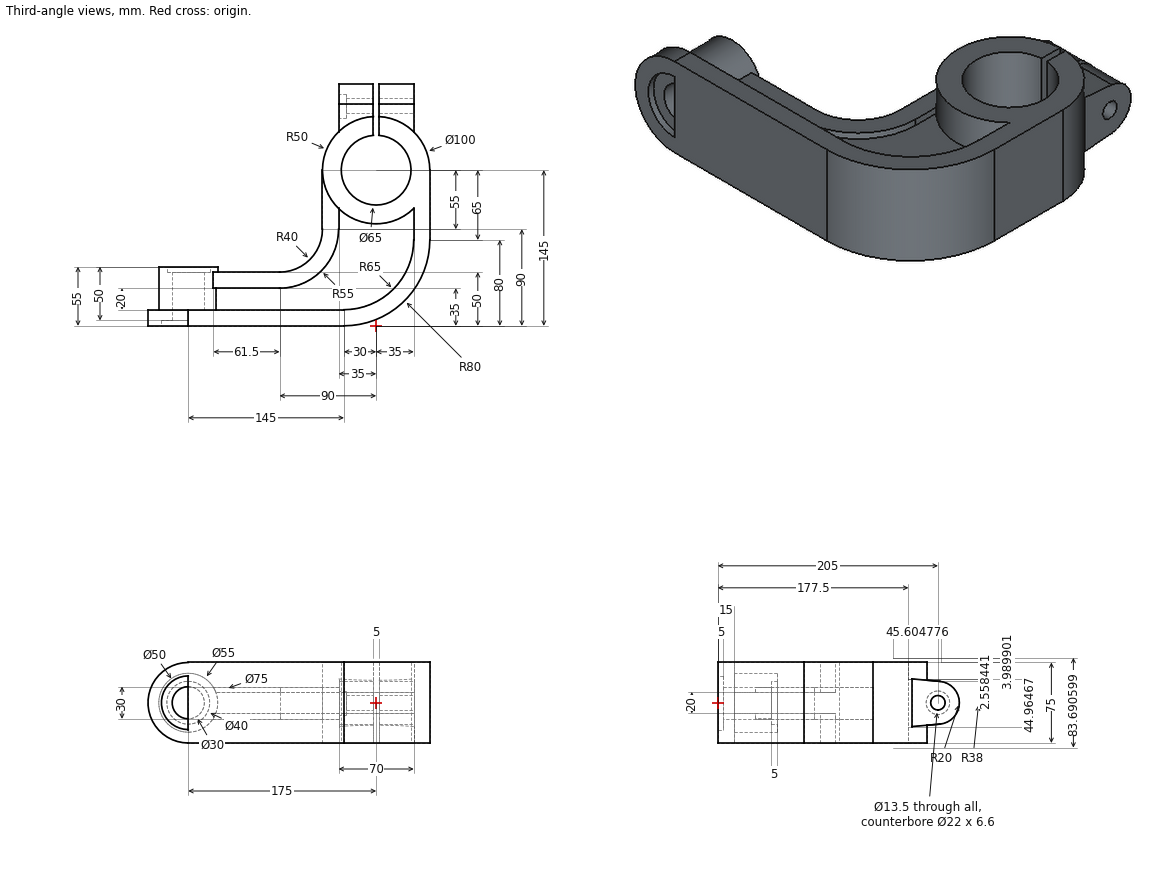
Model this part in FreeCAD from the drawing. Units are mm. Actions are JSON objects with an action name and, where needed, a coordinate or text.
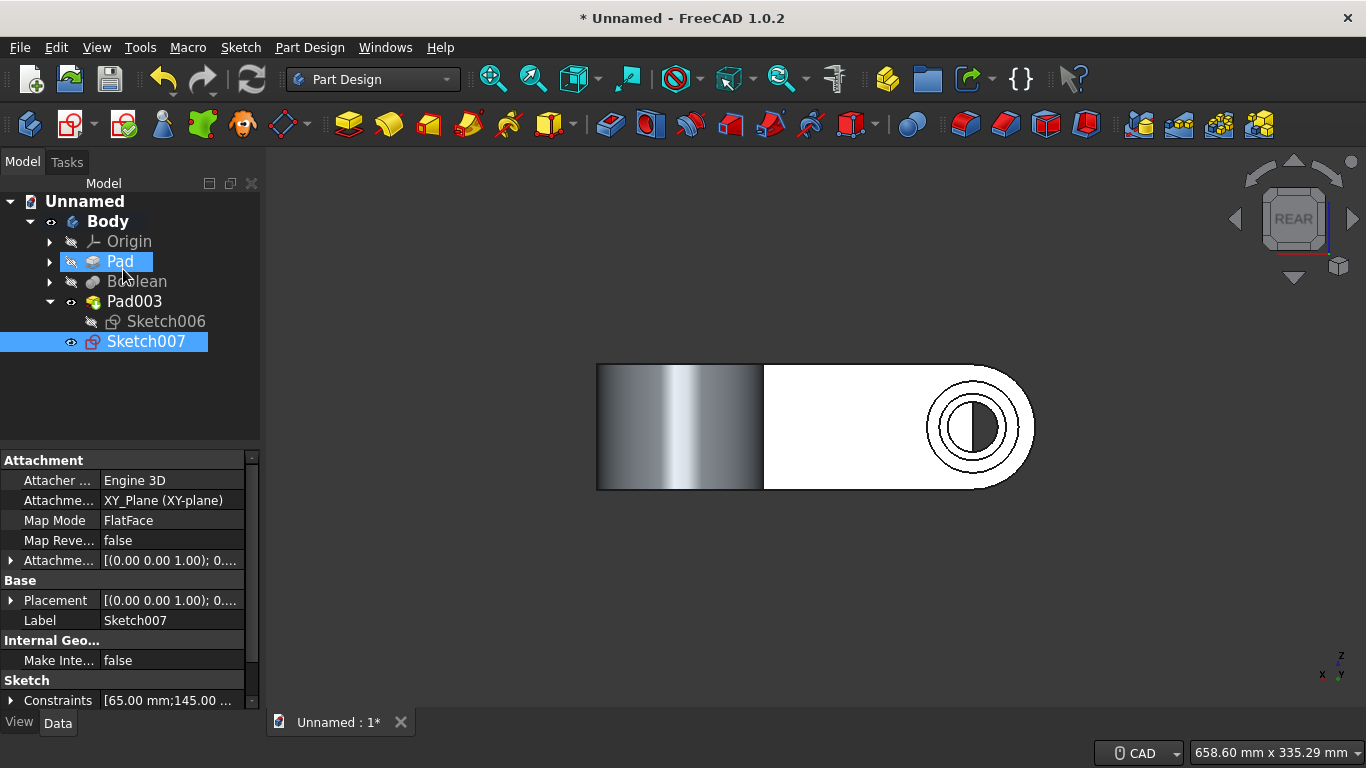
{"action": "left_click", "coordinate": [612, 124]}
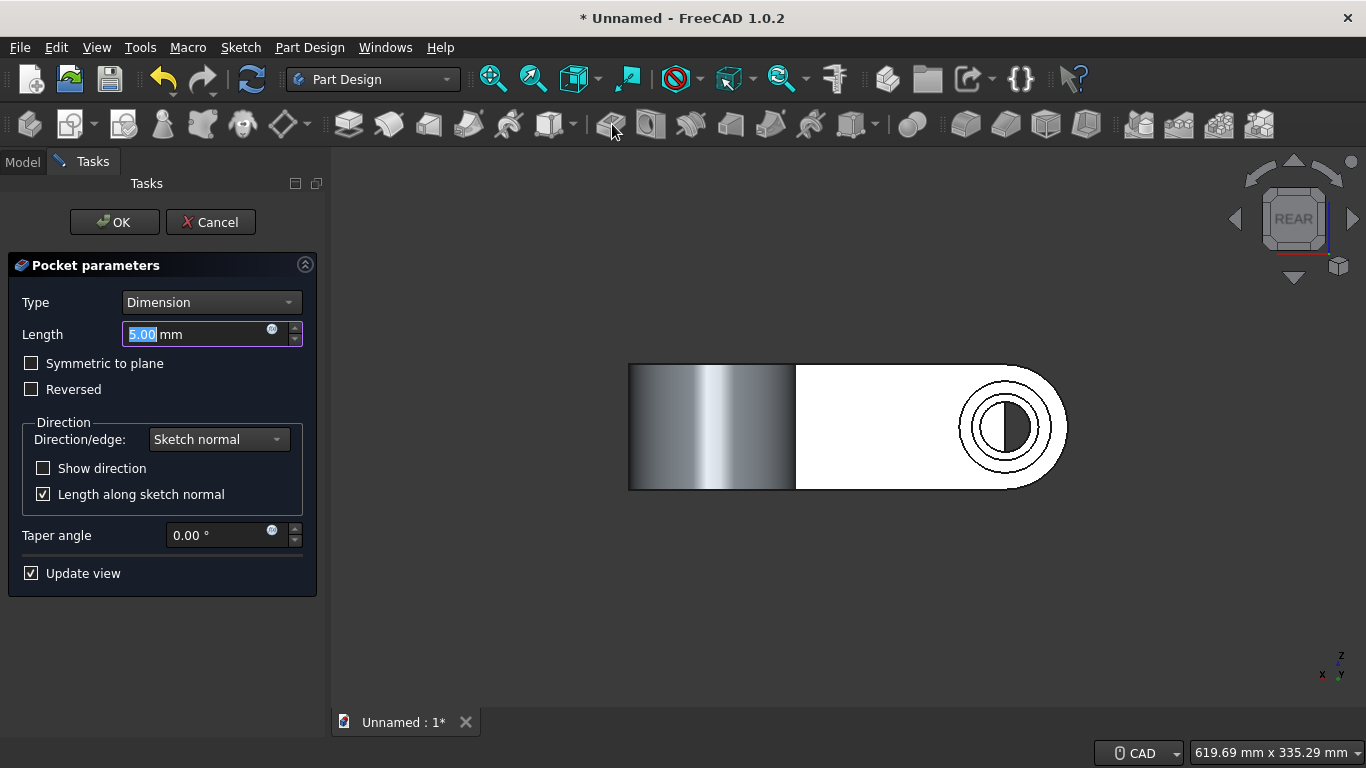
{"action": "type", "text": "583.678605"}
{"action": "key", "text": "Tab"}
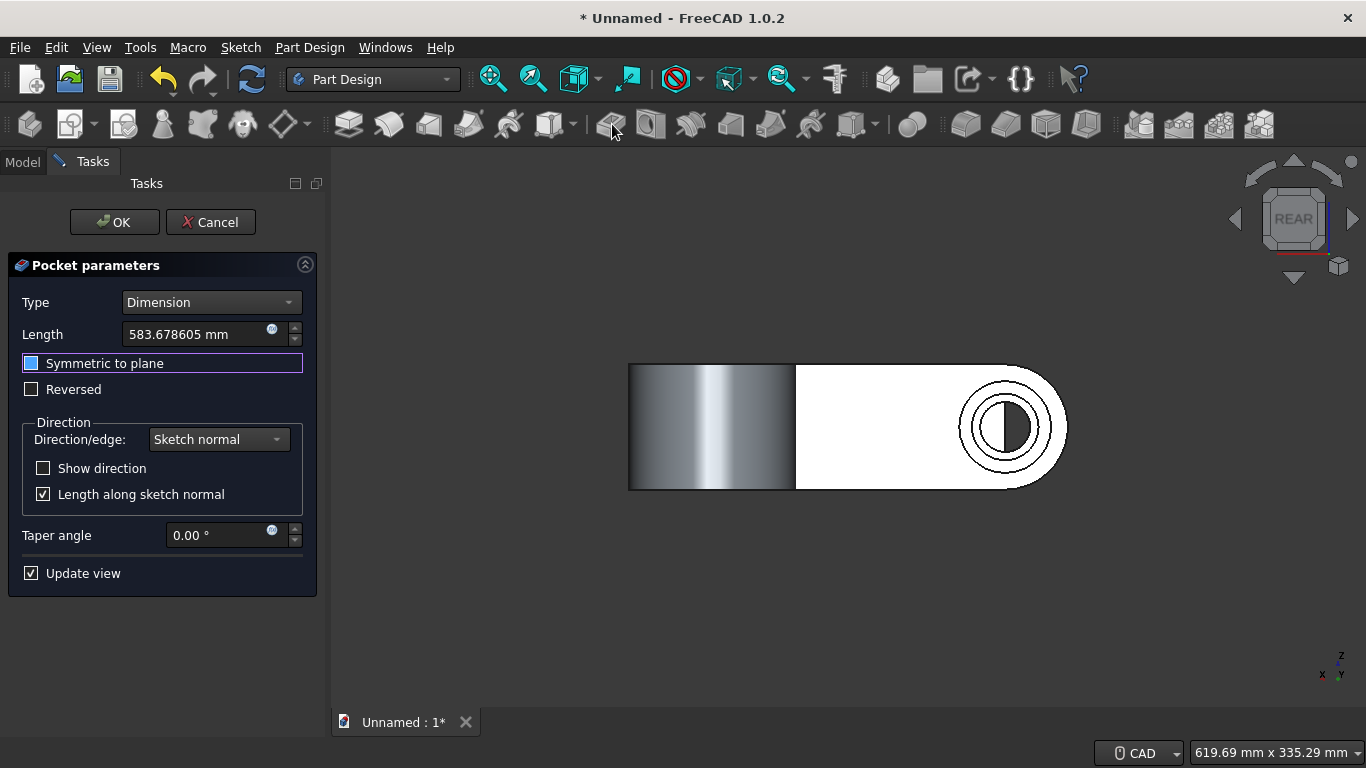
{"action": "left_click", "coordinate": [30, 363]}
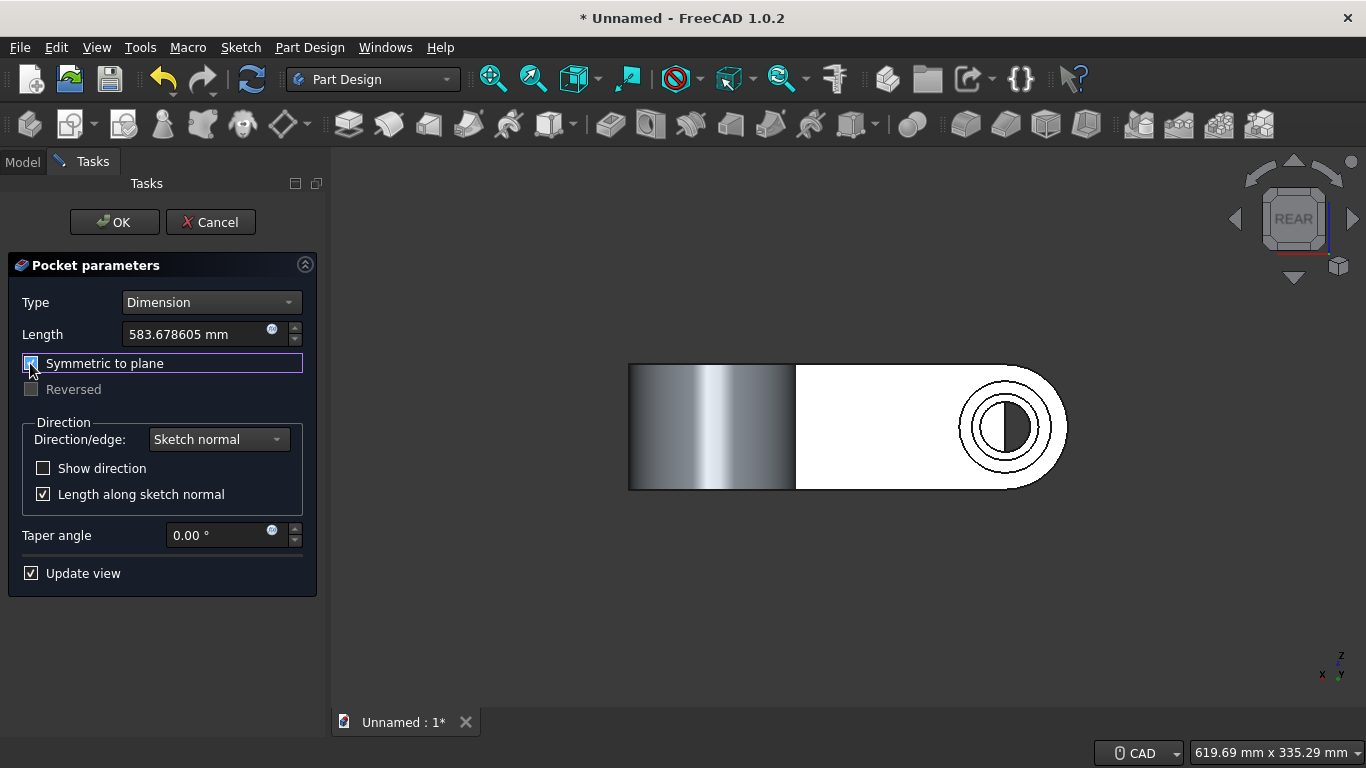
{"action": "left_click", "coordinate": [115, 222]}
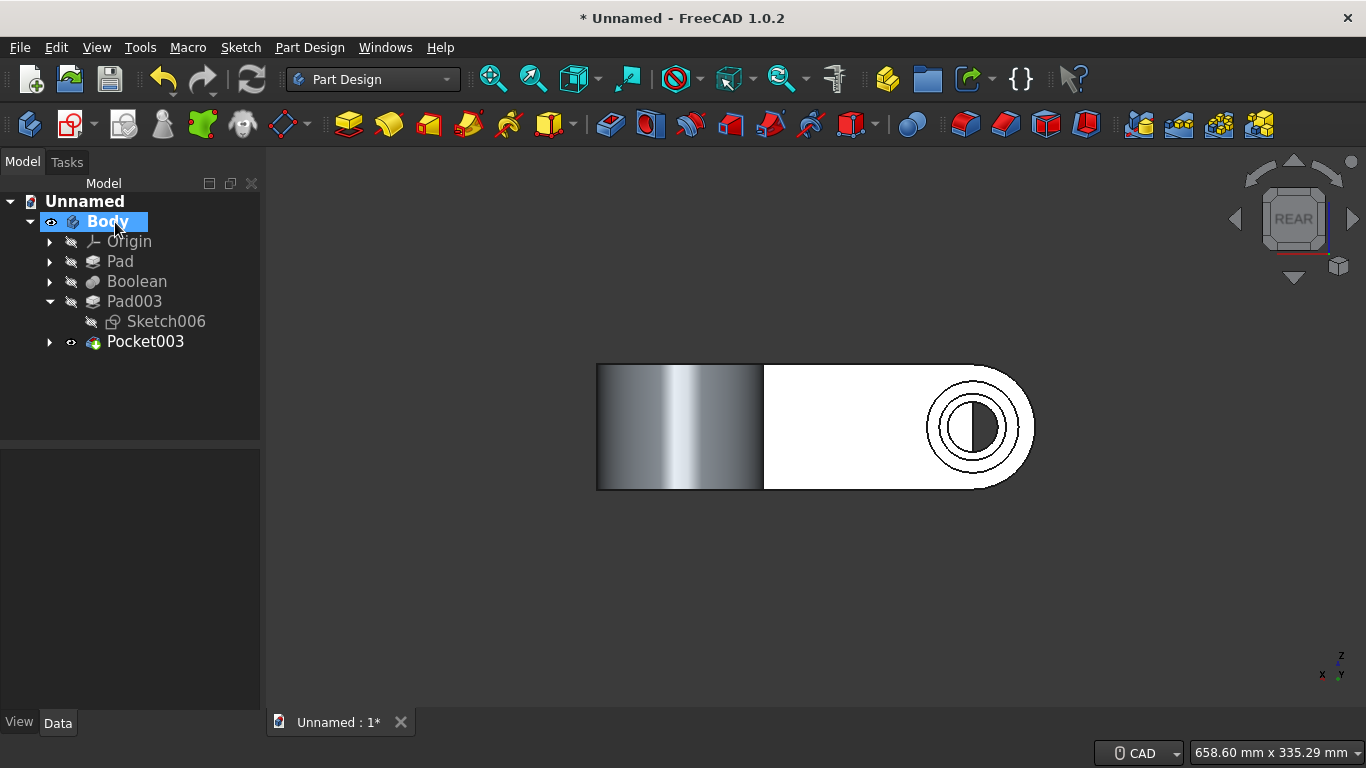
{"action": "key", "text": "v f"}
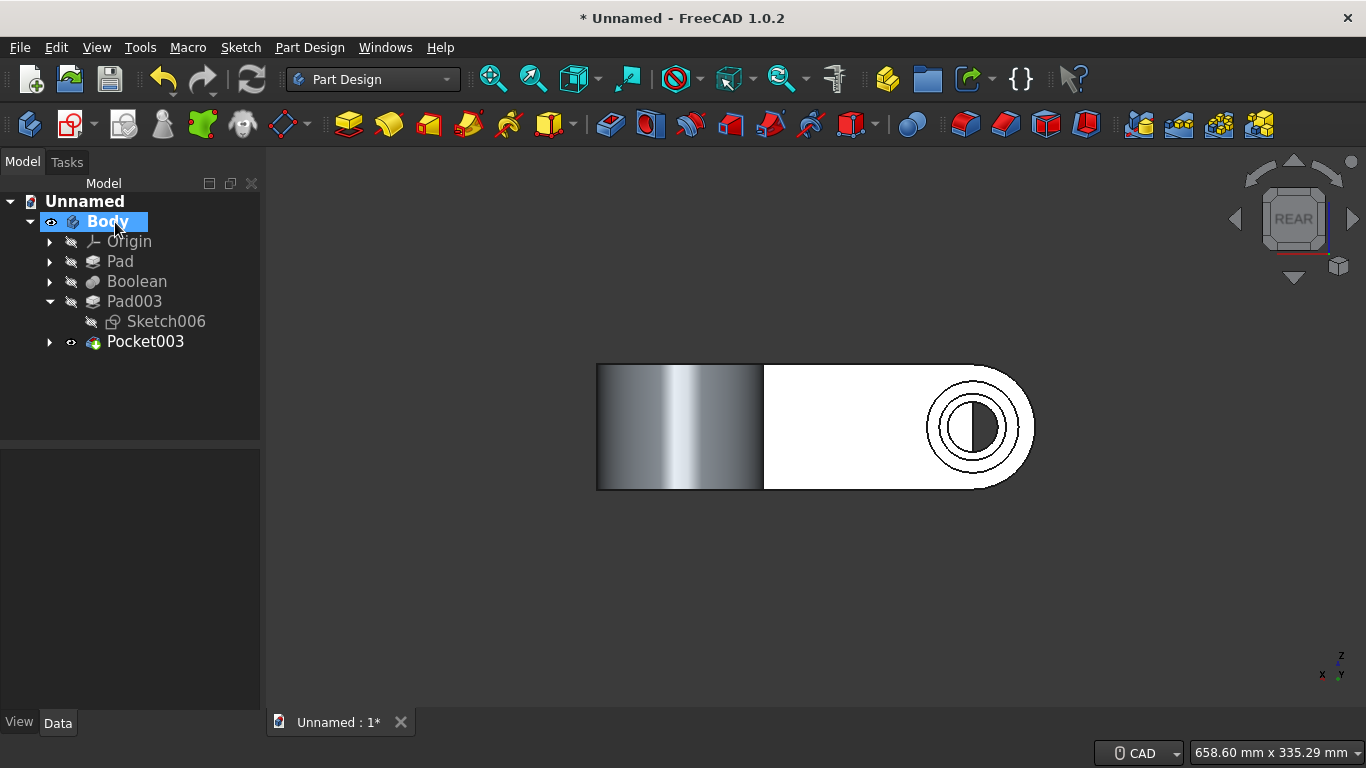
{"action": "left_click", "coordinate": [70, 124]}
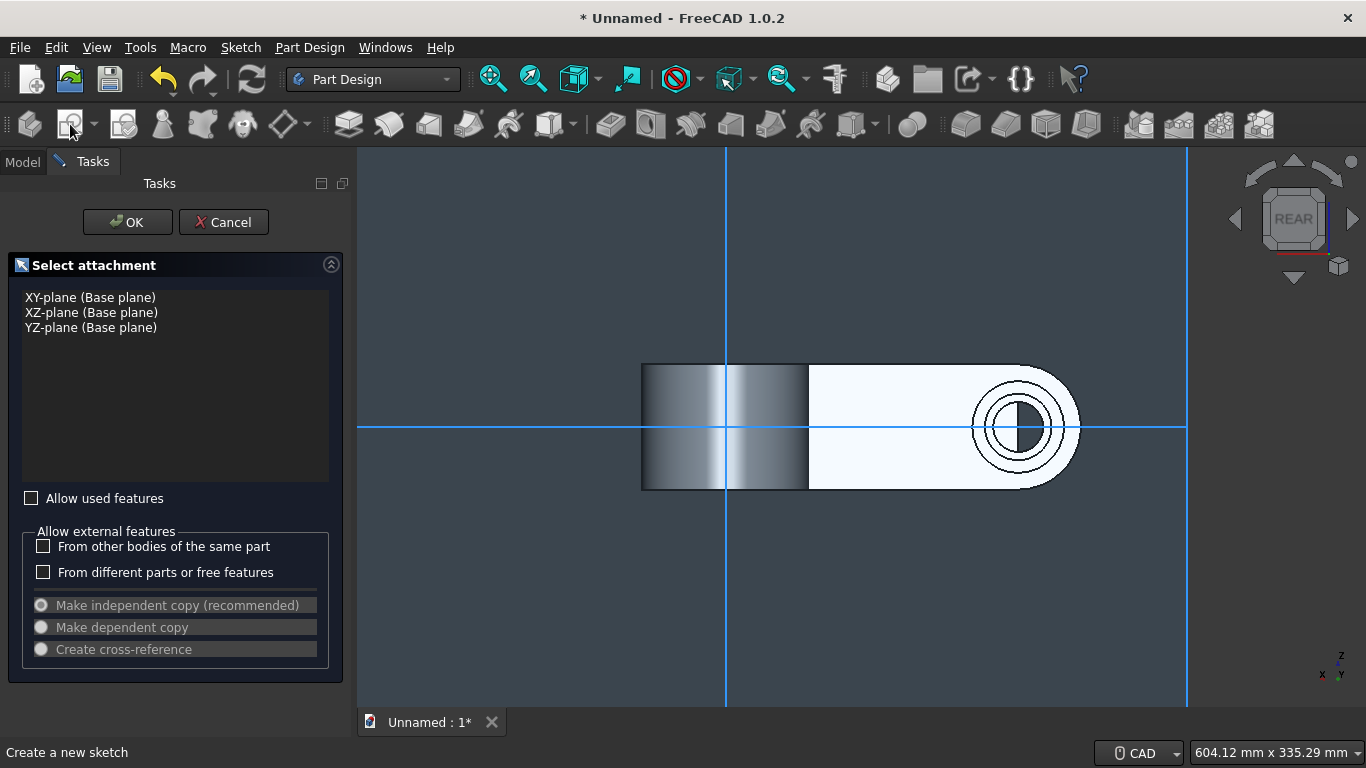
{"action": "left_click", "coordinate": [82, 298]}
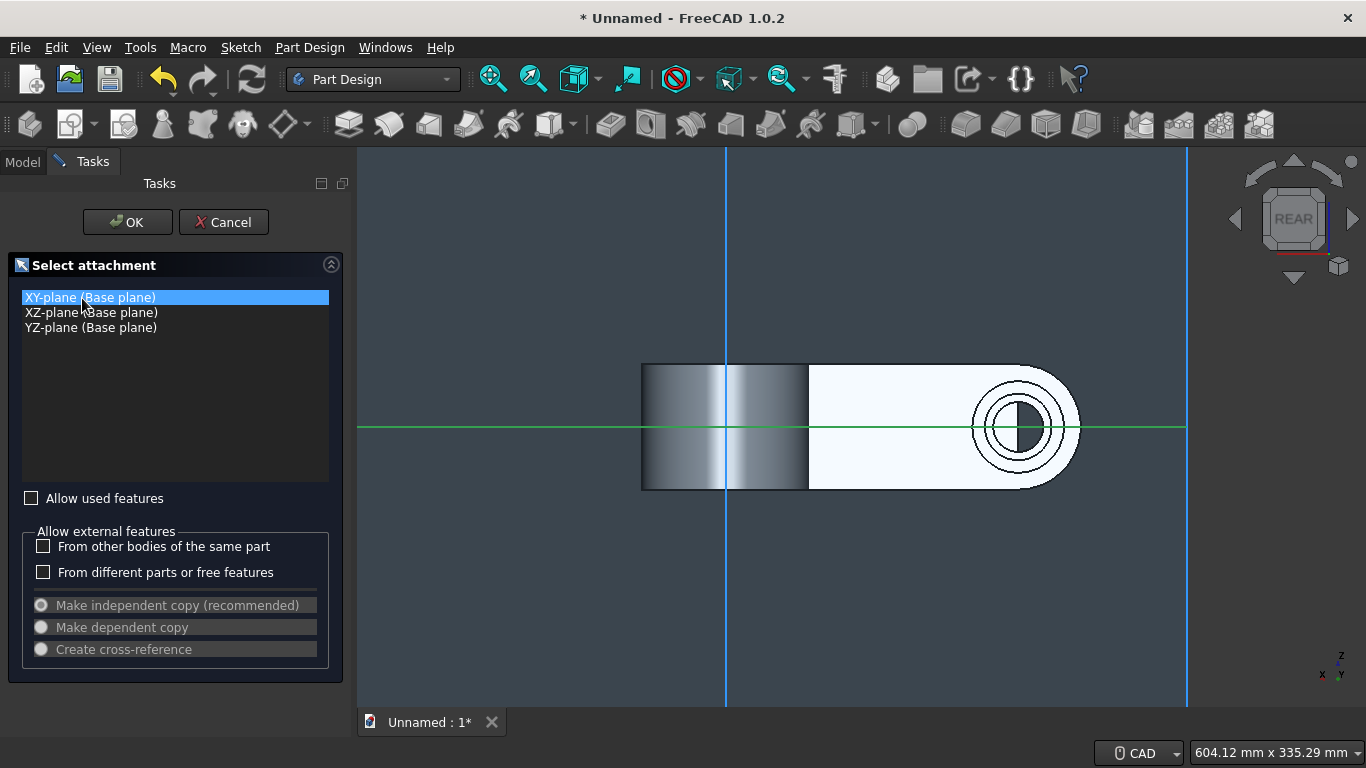
{"action": "left_click", "coordinate": [128, 222]}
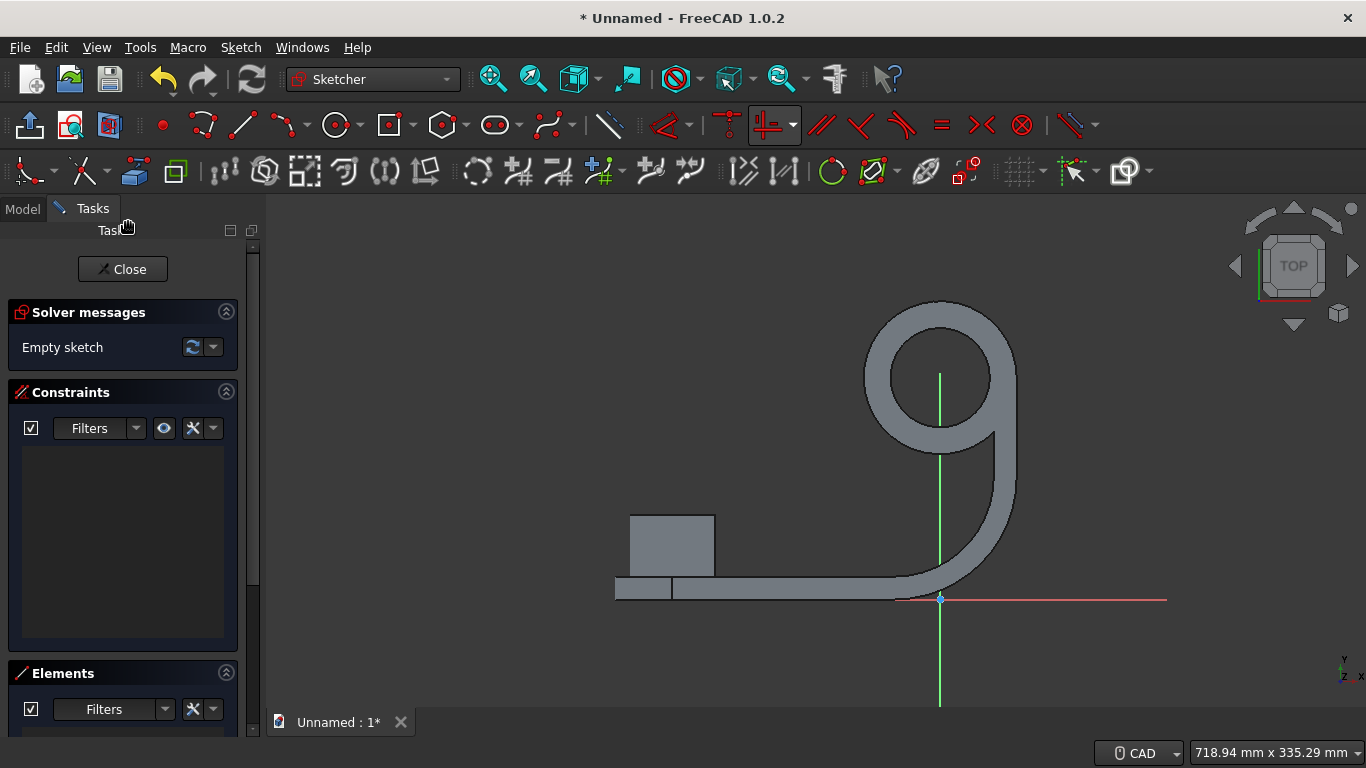
{"action": "key", "text": "q s"}